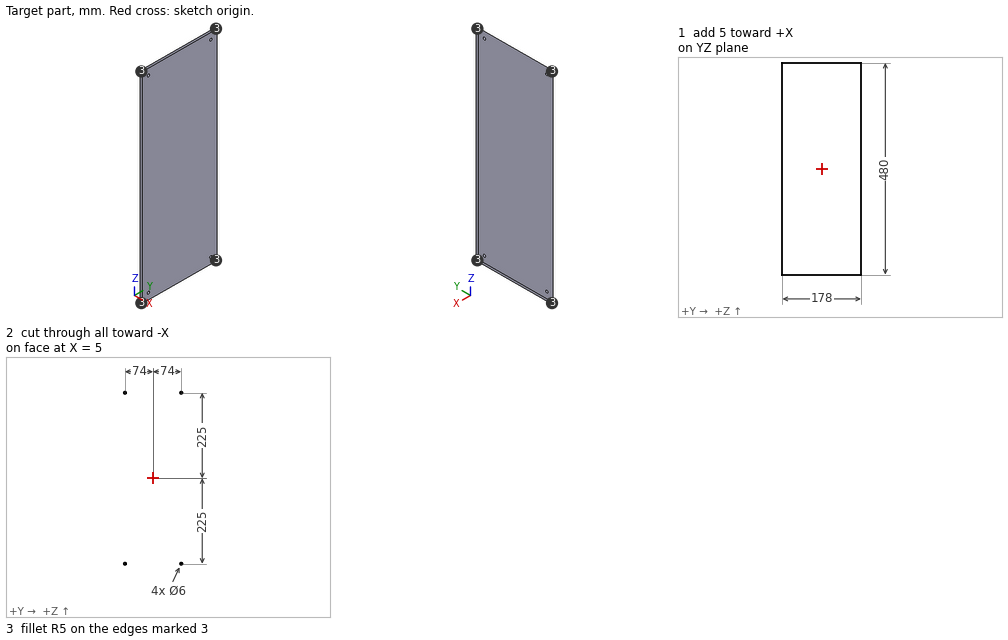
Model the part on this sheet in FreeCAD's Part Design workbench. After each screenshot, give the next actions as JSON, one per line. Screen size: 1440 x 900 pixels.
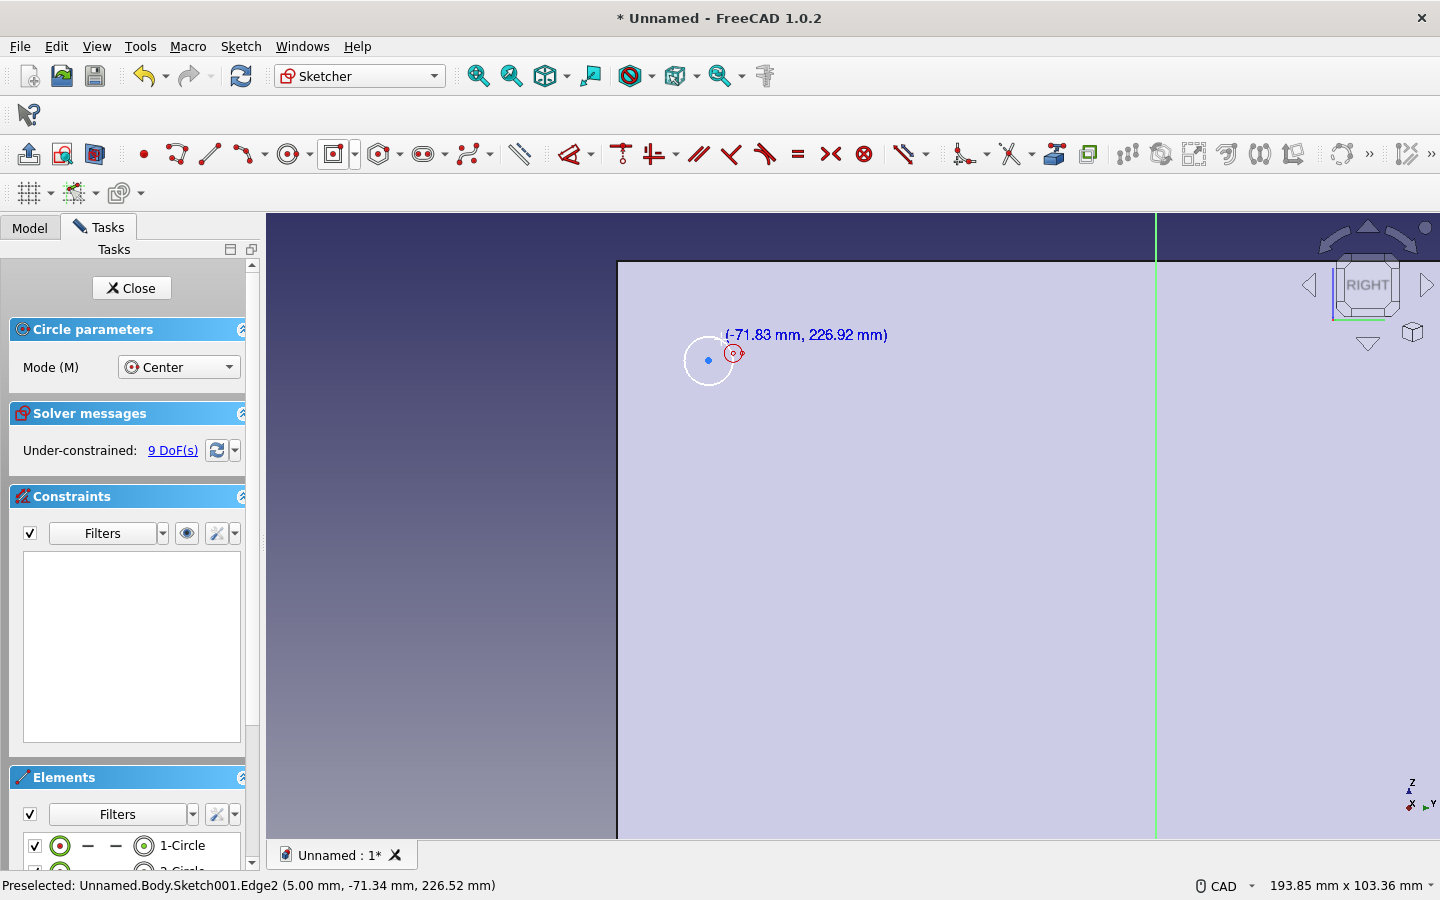
{"action": "scroll", "coordinate": [726, 340], "scroll_direction": "down", "scroll_amount": 10}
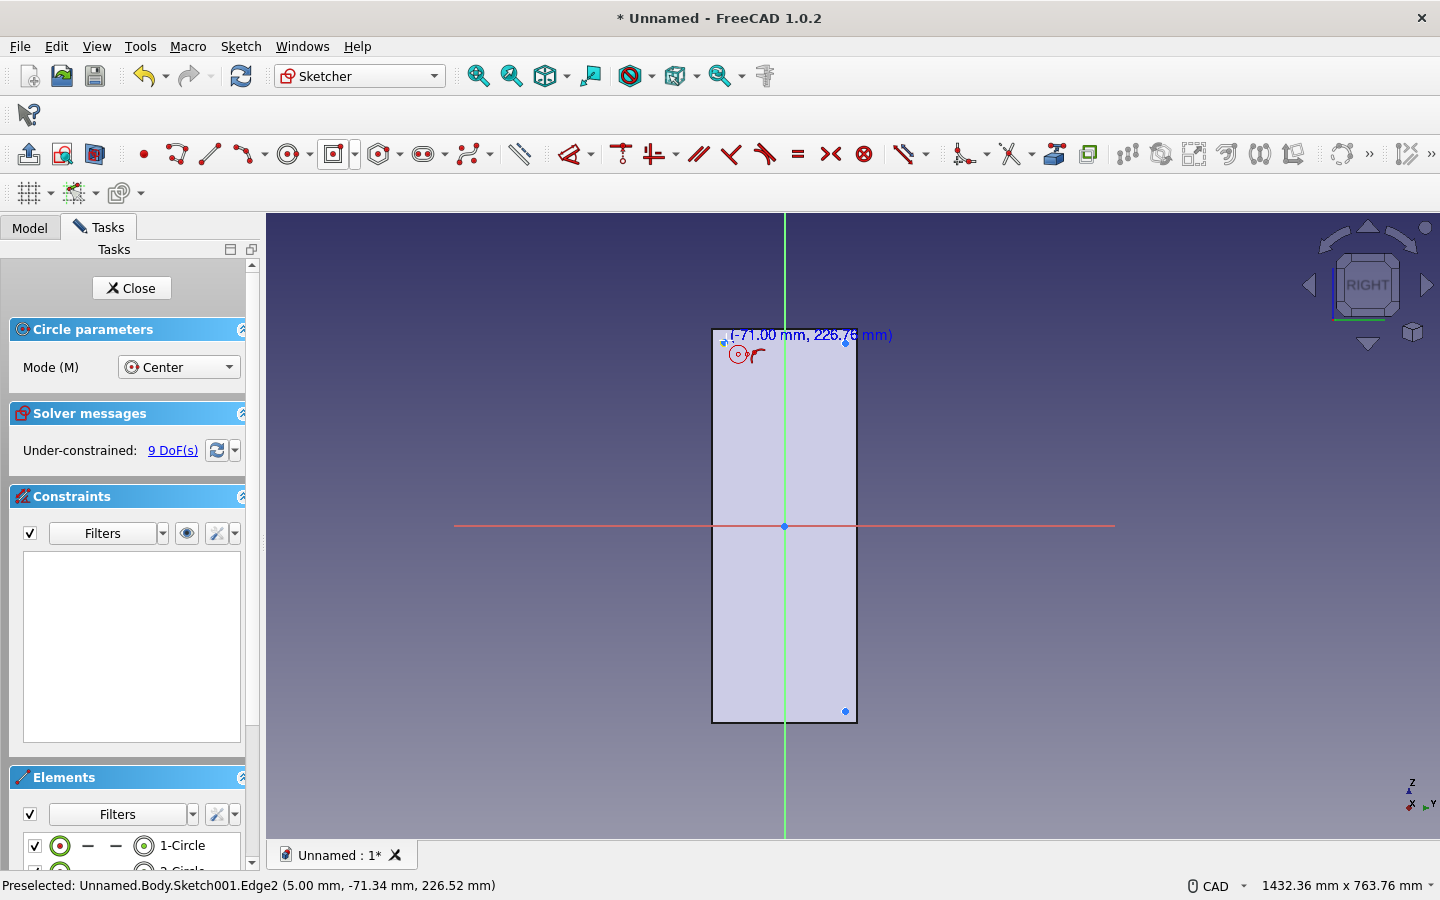
{"action": "scroll", "coordinate": [724, 711], "scroll_direction": "up", "scroll_amount": 12}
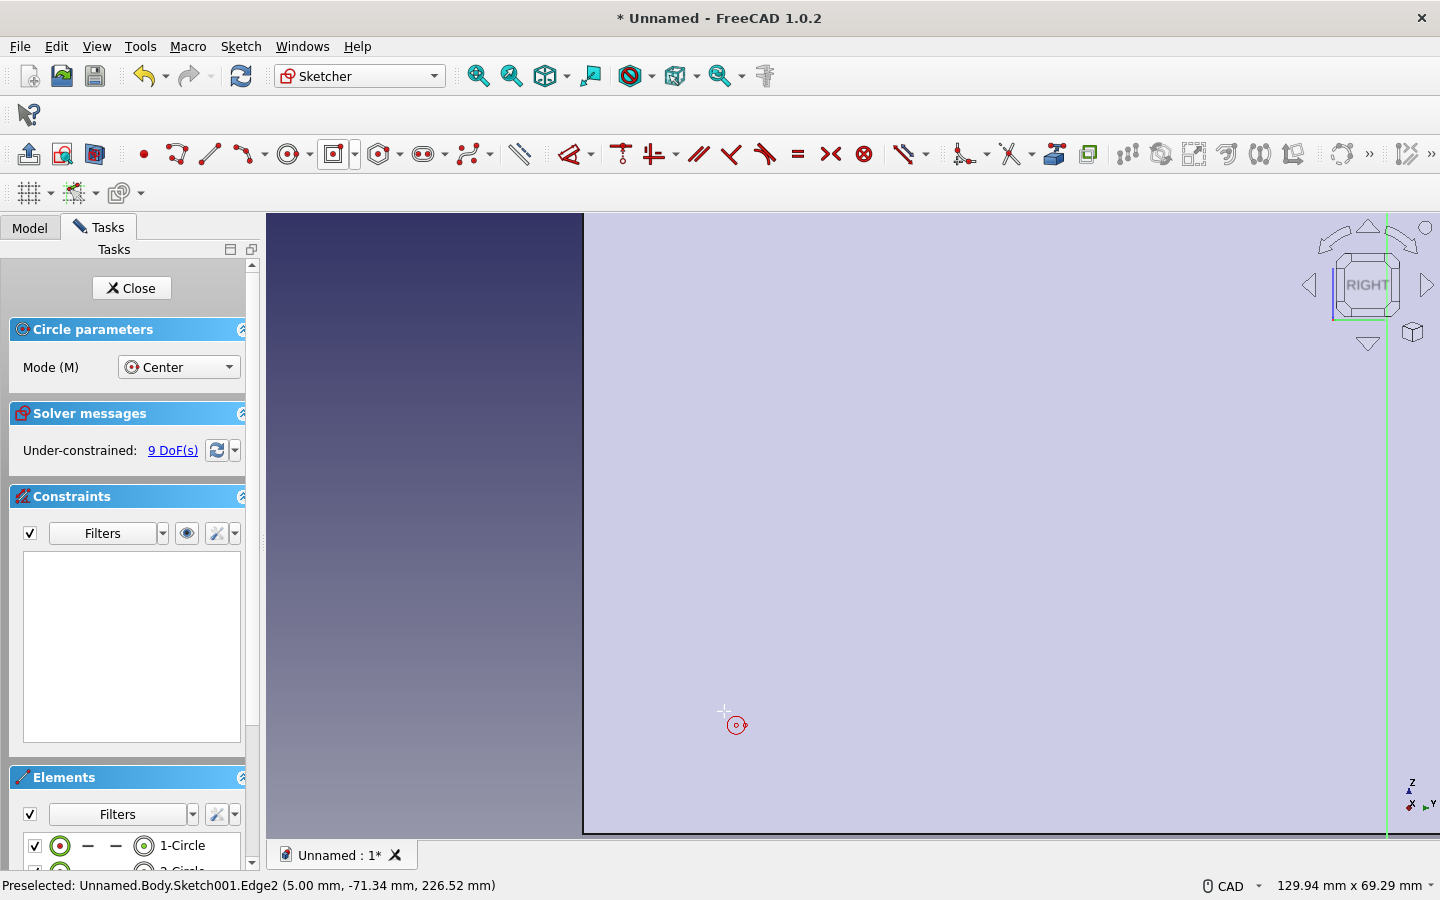
{"action": "scroll", "coordinate": [724, 712], "scroll_direction": "down", "scroll_amount": 12}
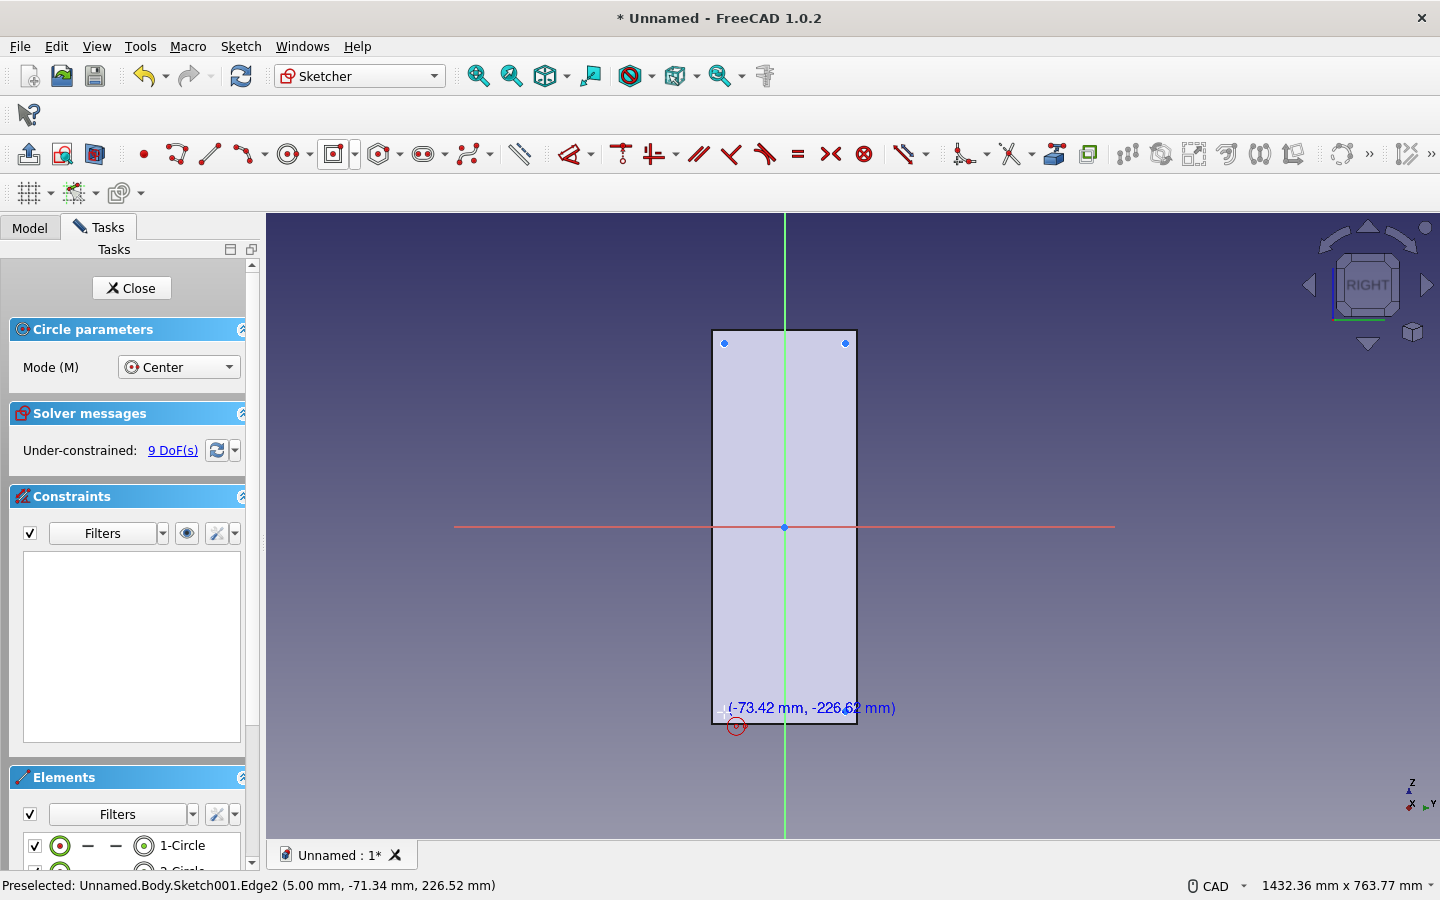
{"action": "left_click", "coordinate": [724, 711]}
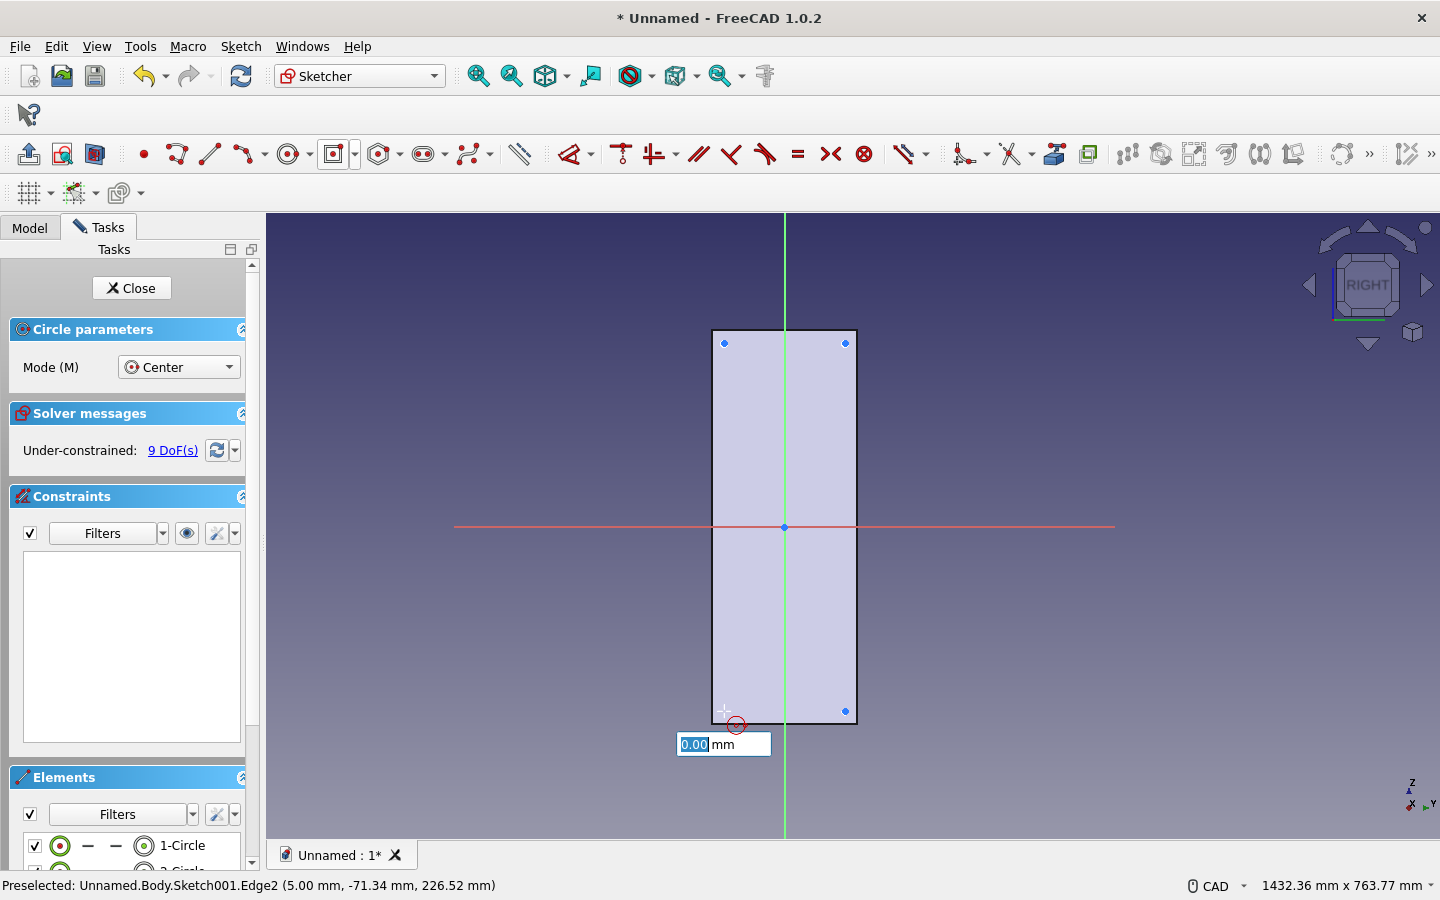
{"action": "scroll", "coordinate": [726, 710], "scroll_direction": "up", "scroll_amount": 10}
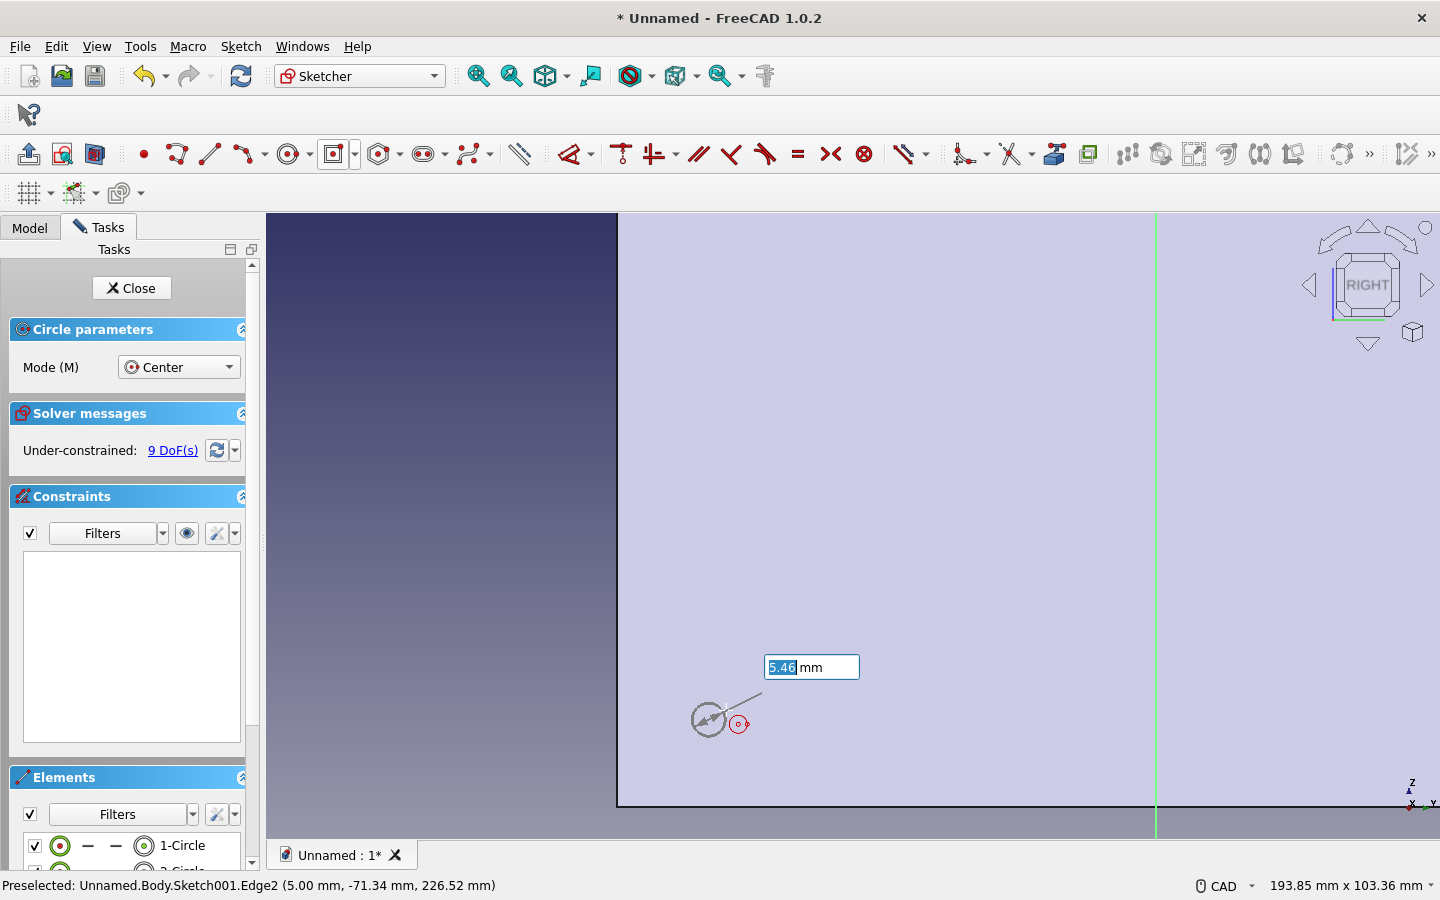
{"action": "left_click", "coordinate": [721, 703]}
{"action": "key", "text": "Escape"}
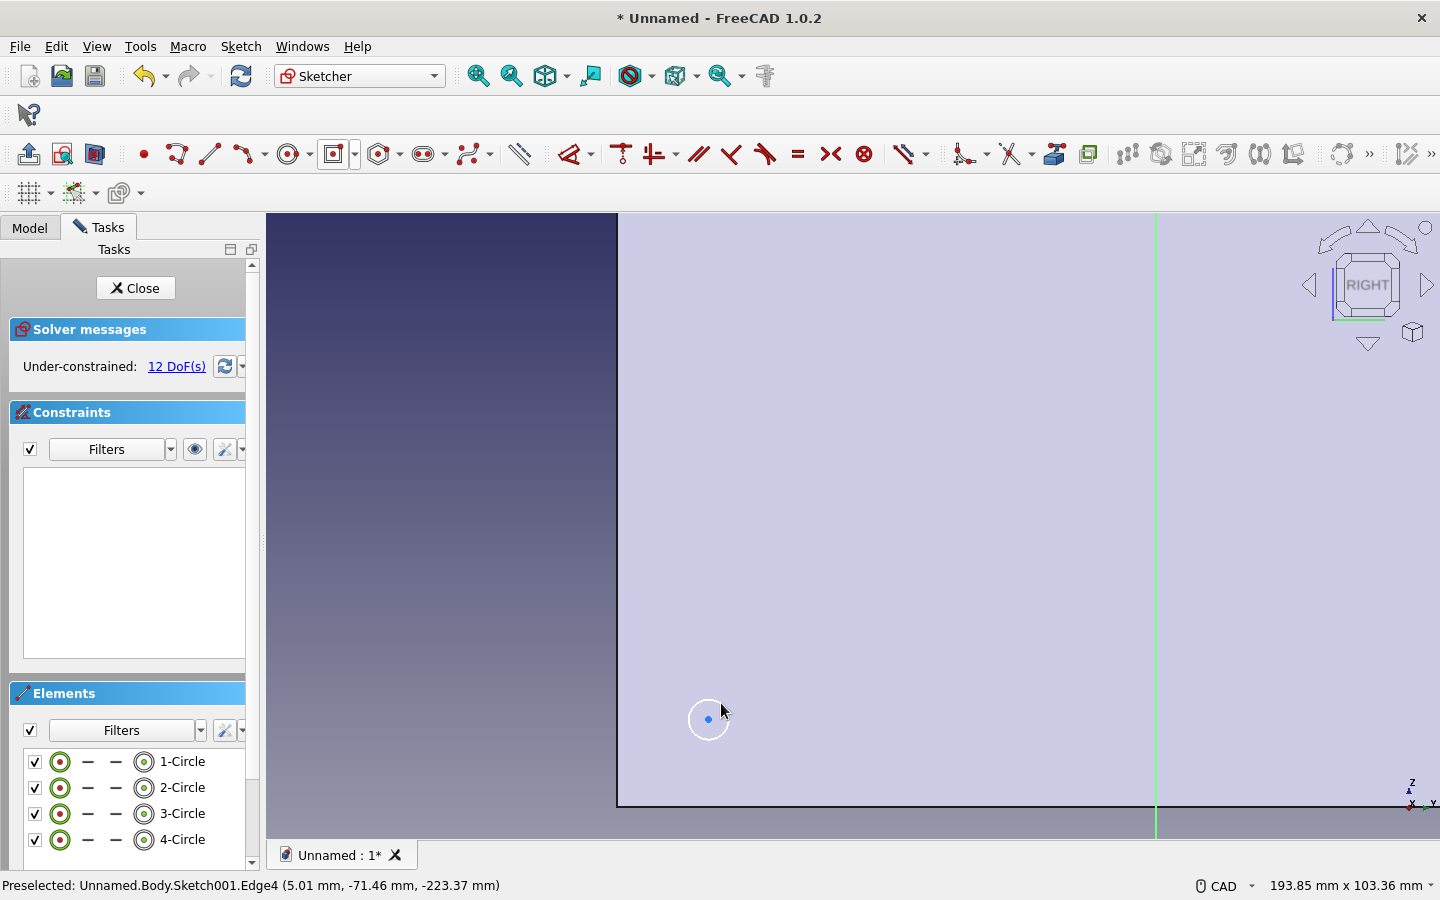
{"action": "scroll", "coordinate": [726, 710], "scroll_direction": "down", "scroll_amount": 10}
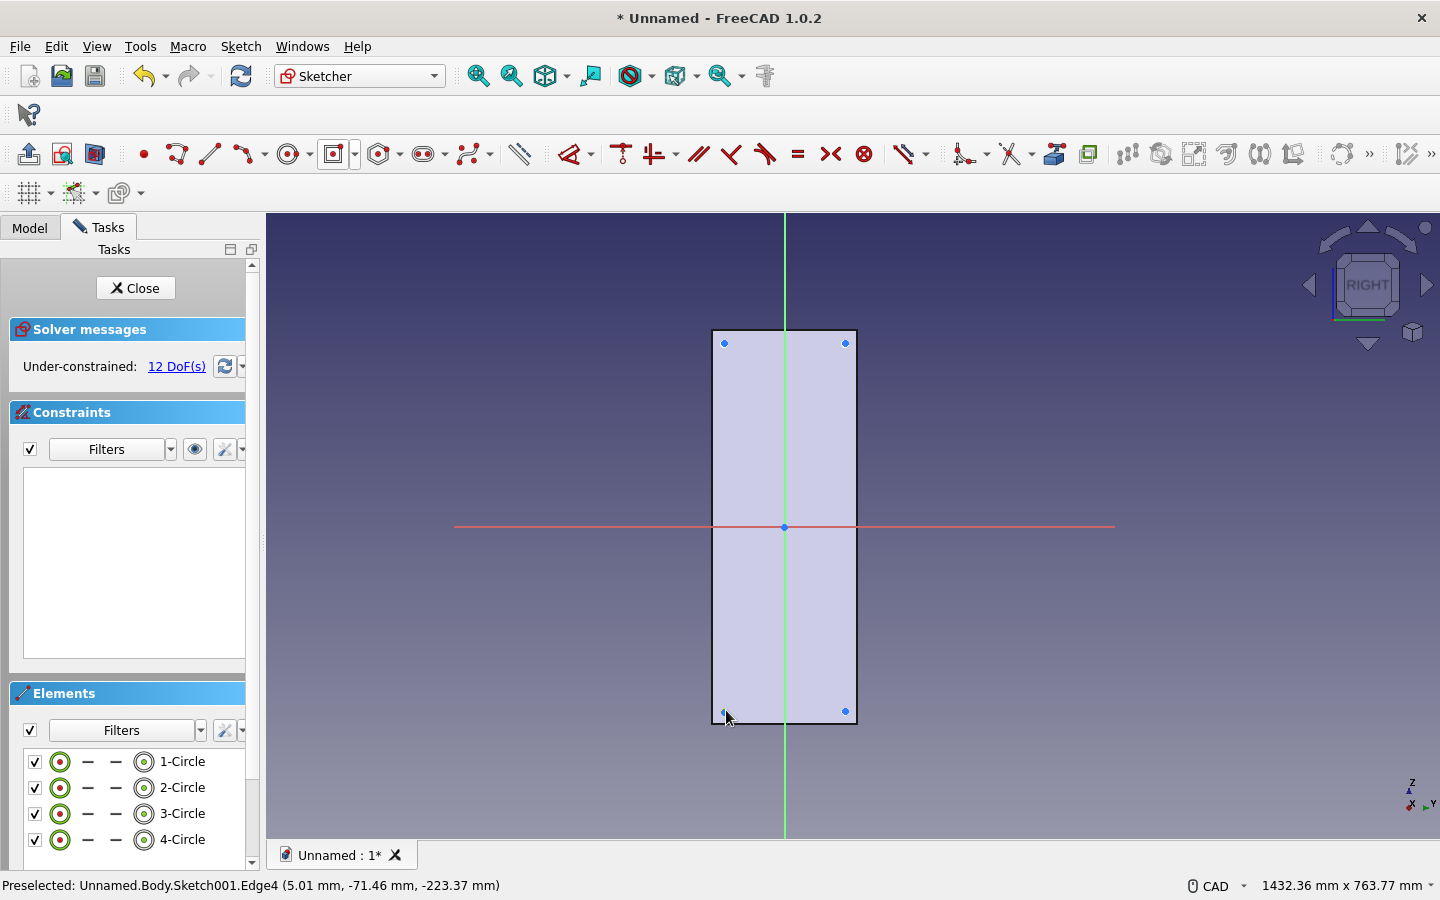
{"action": "scroll", "coordinate": [847, 342], "scroll_direction": "up", "scroll_amount": 8}